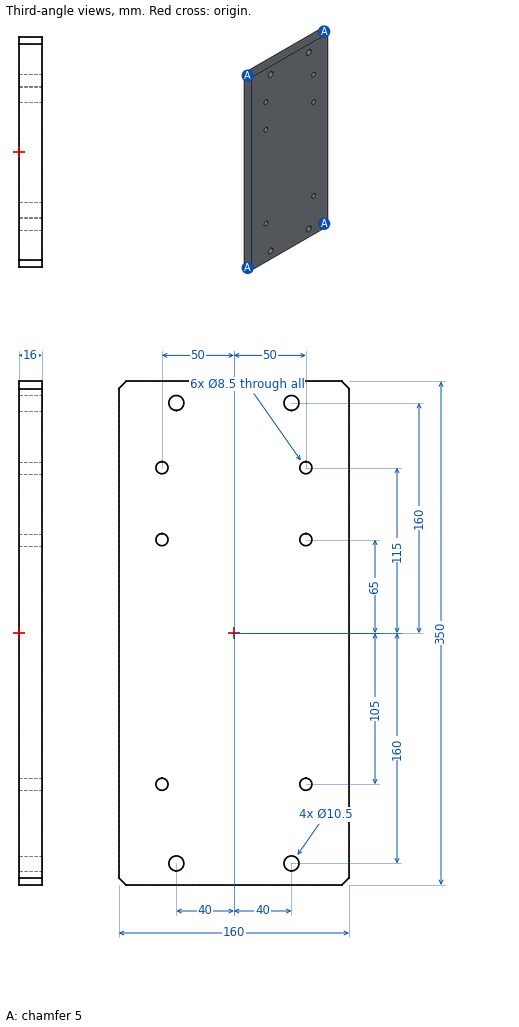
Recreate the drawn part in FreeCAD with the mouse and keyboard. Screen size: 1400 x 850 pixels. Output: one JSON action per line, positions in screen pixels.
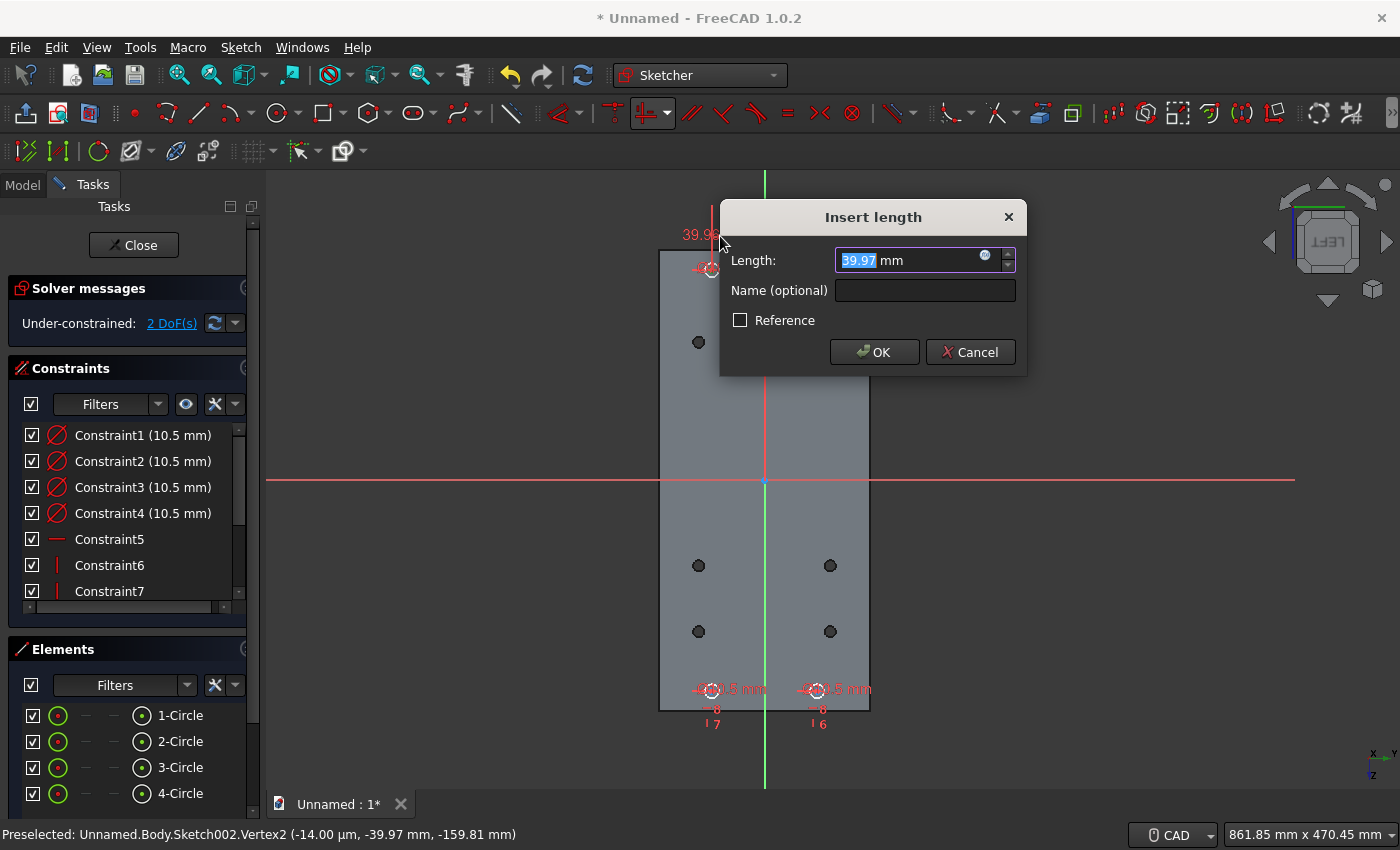
{"action": "type", "text": "40"}
{"action": "key", "text": "Return"}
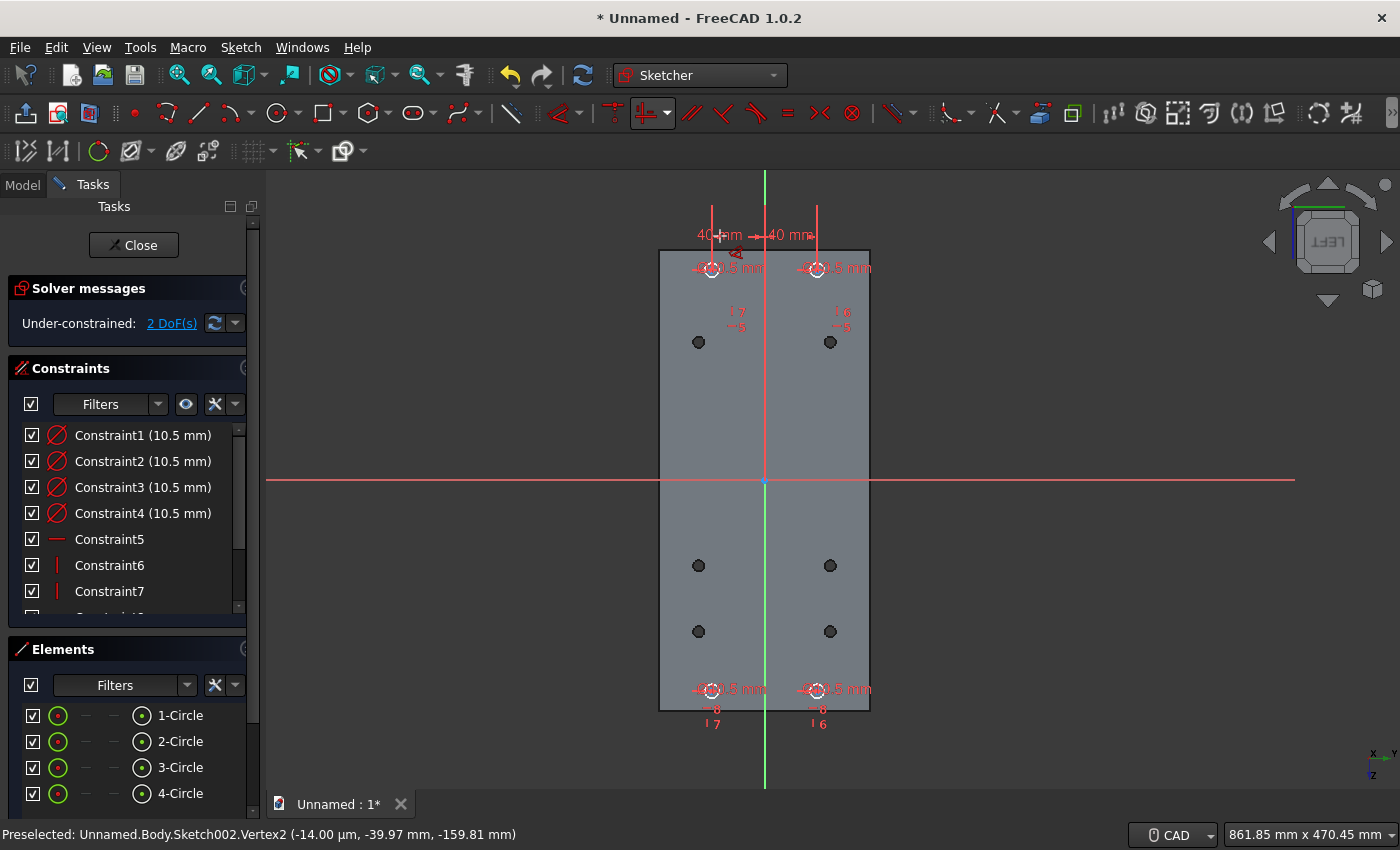
{"action": "left_click", "coordinate": [817, 270]}
{"action": "left_click", "coordinate": [851, 375]}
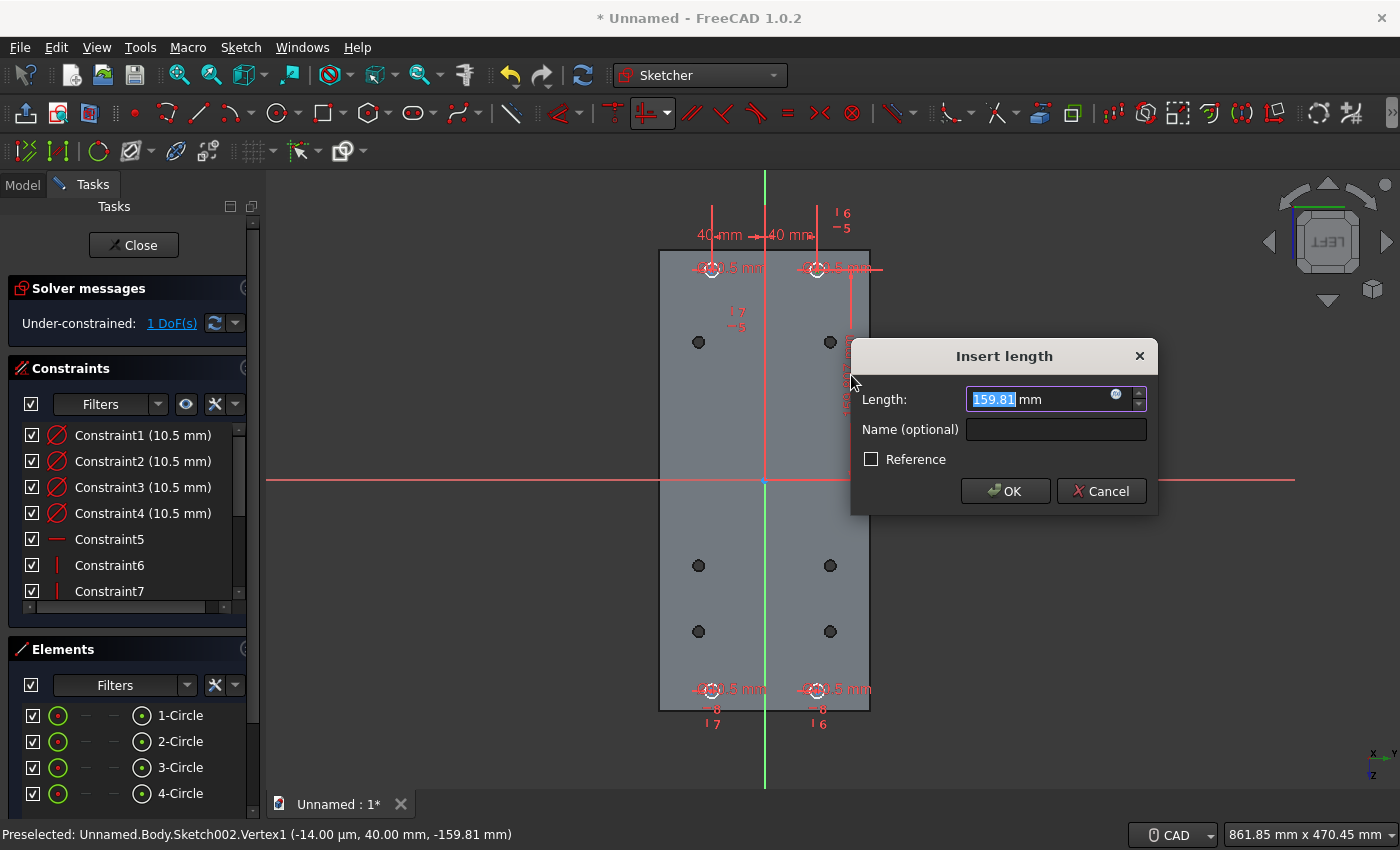
{"action": "type", "text": "160"}
{"action": "key", "text": "Return"}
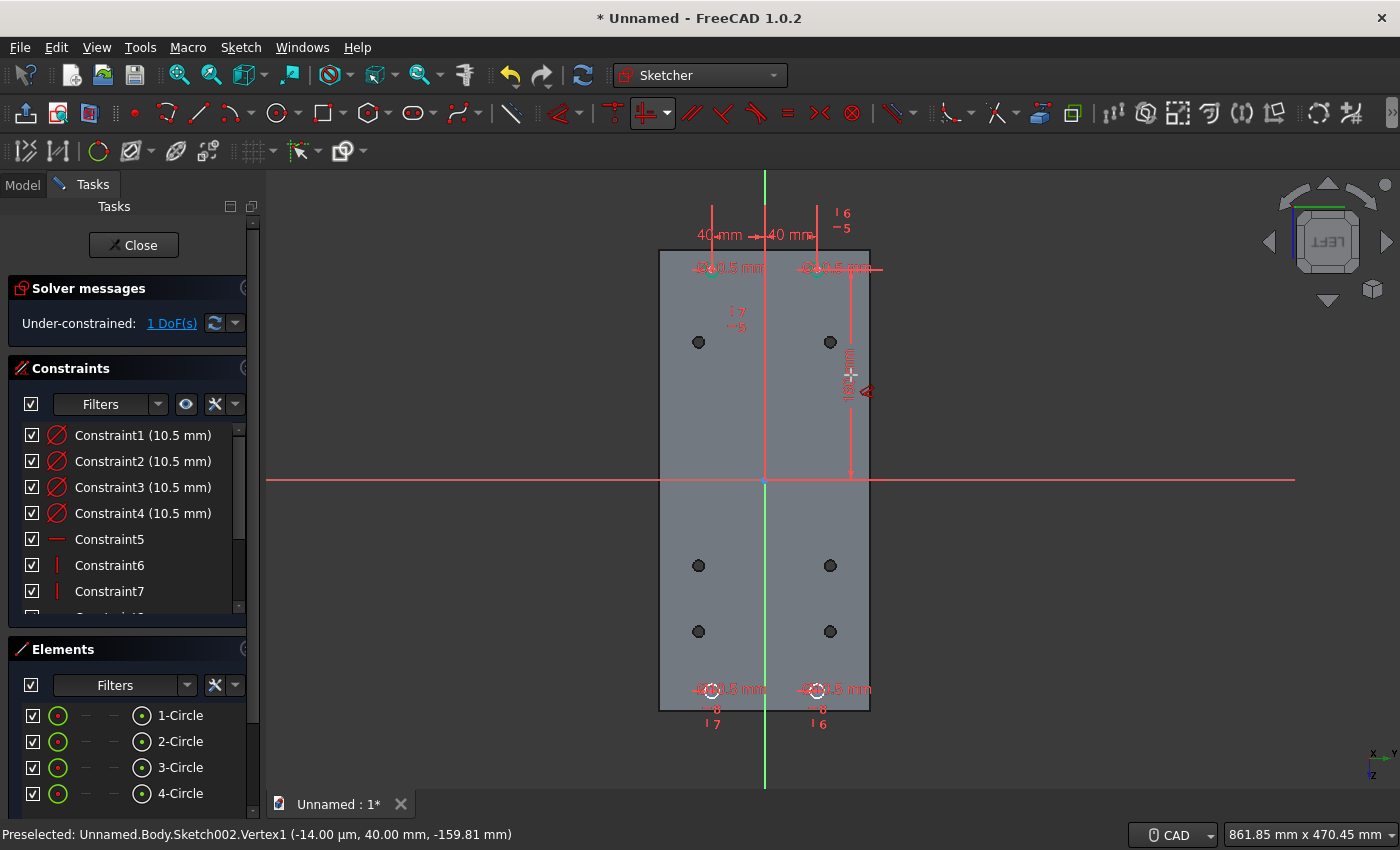
{"action": "left_click", "coordinate": [817, 691]}
{"action": "left_click", "coordinate": [851, 586]}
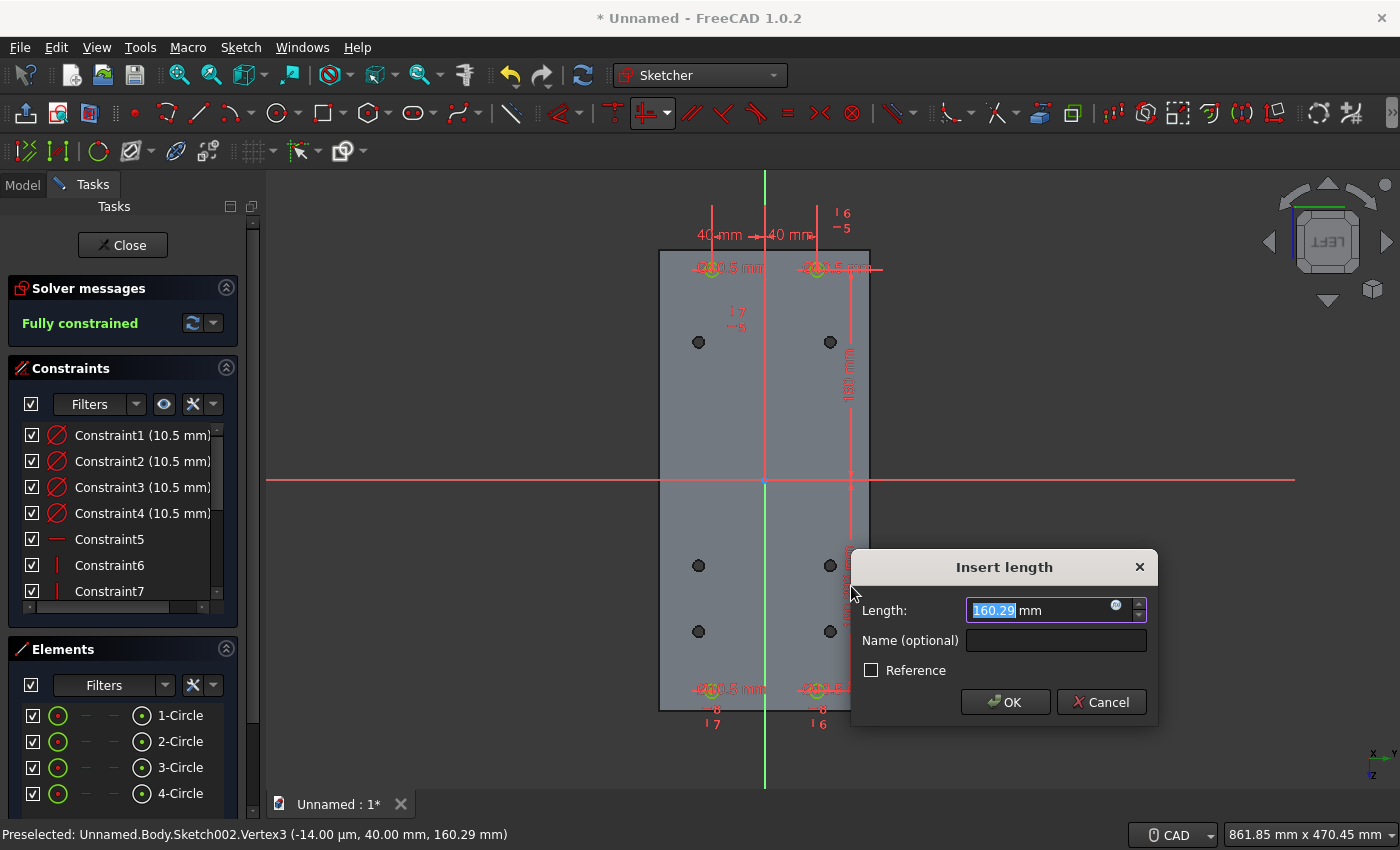
{"action": "type", "text": "160"}
{"action": "key", "text": "Return"}
{"action": "key", "text": "Escape"}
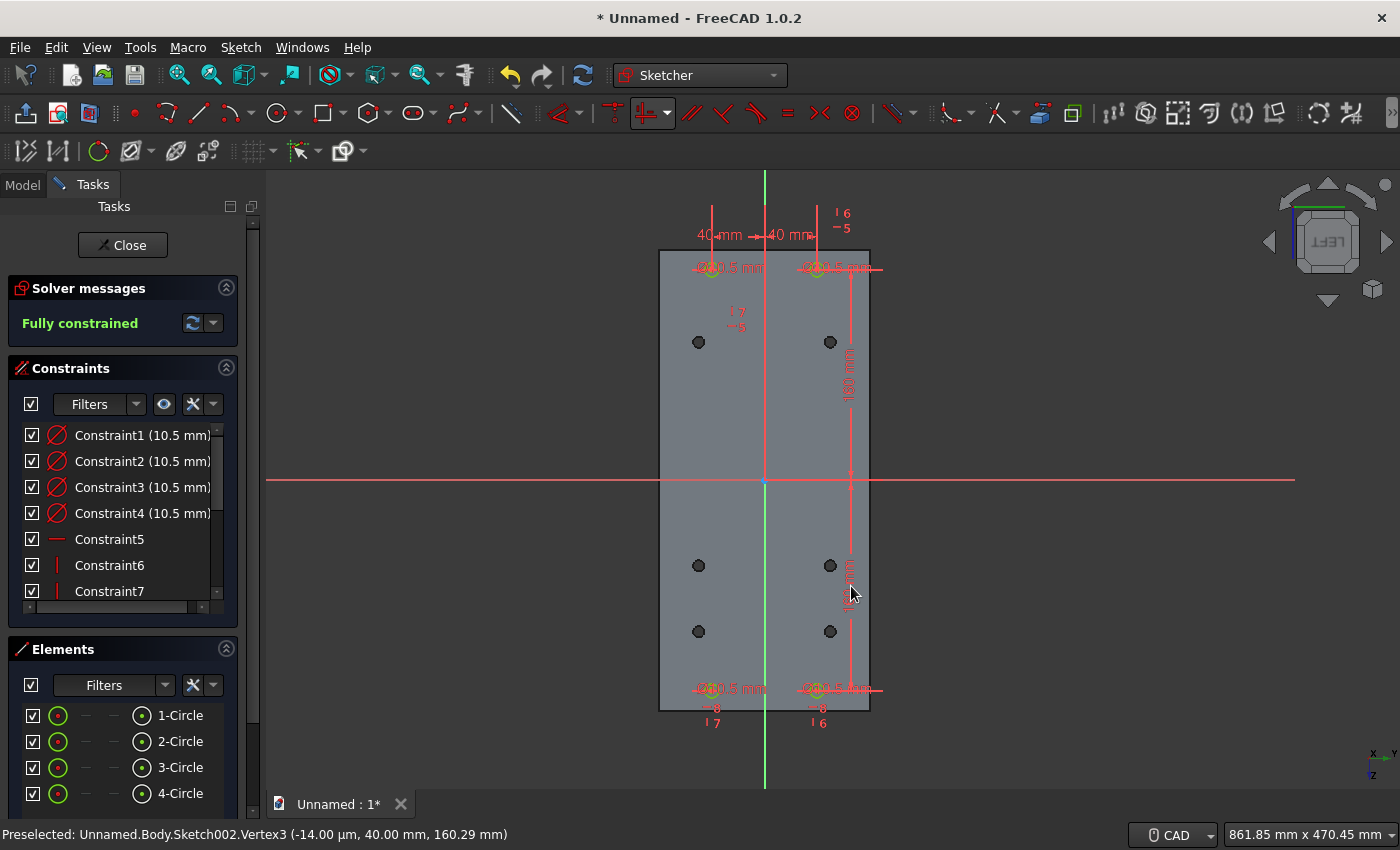
{"action": "left_click", "coordinate": [123, 245]}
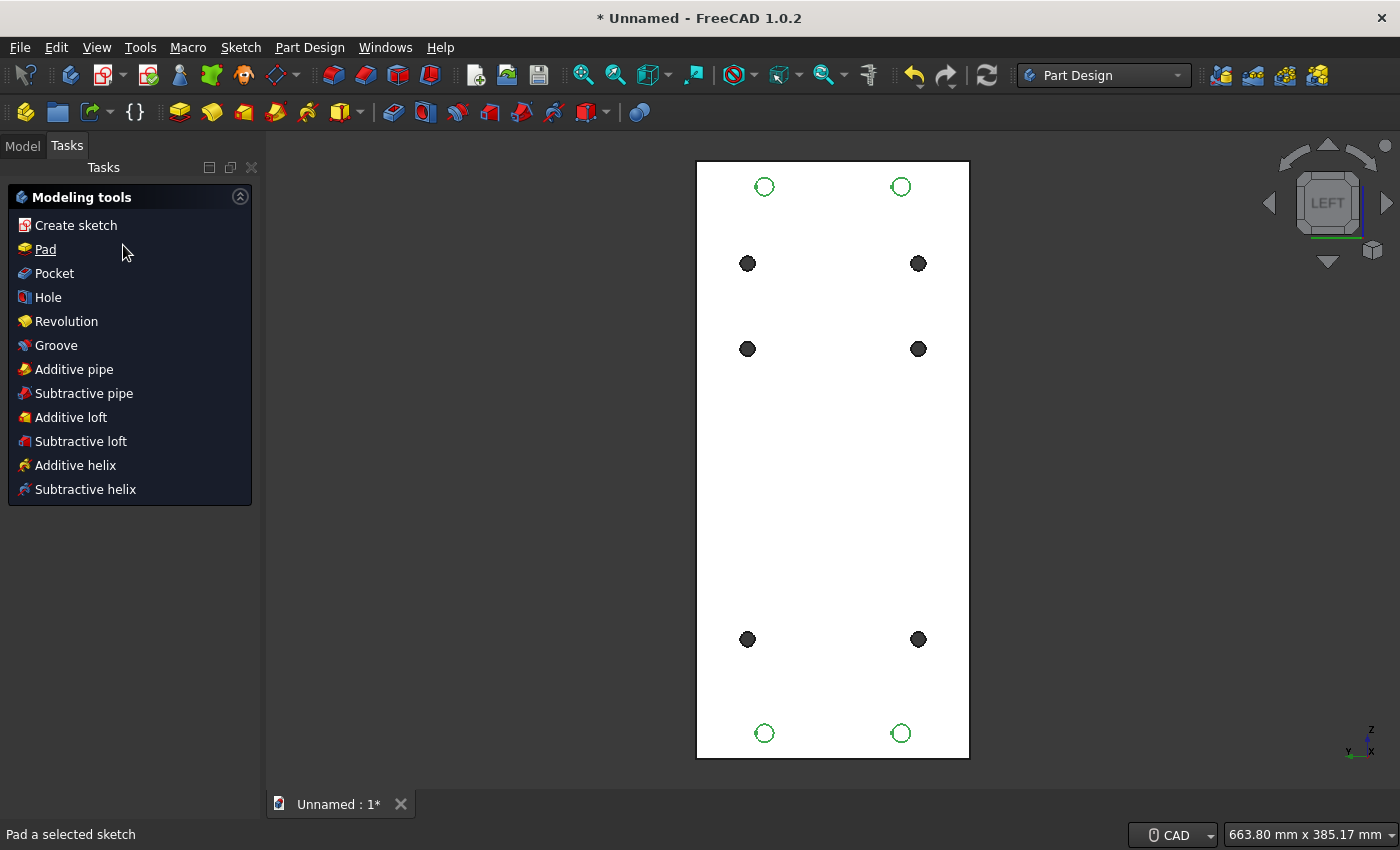
{"action": "left_click", "coordinate": [394, 112]}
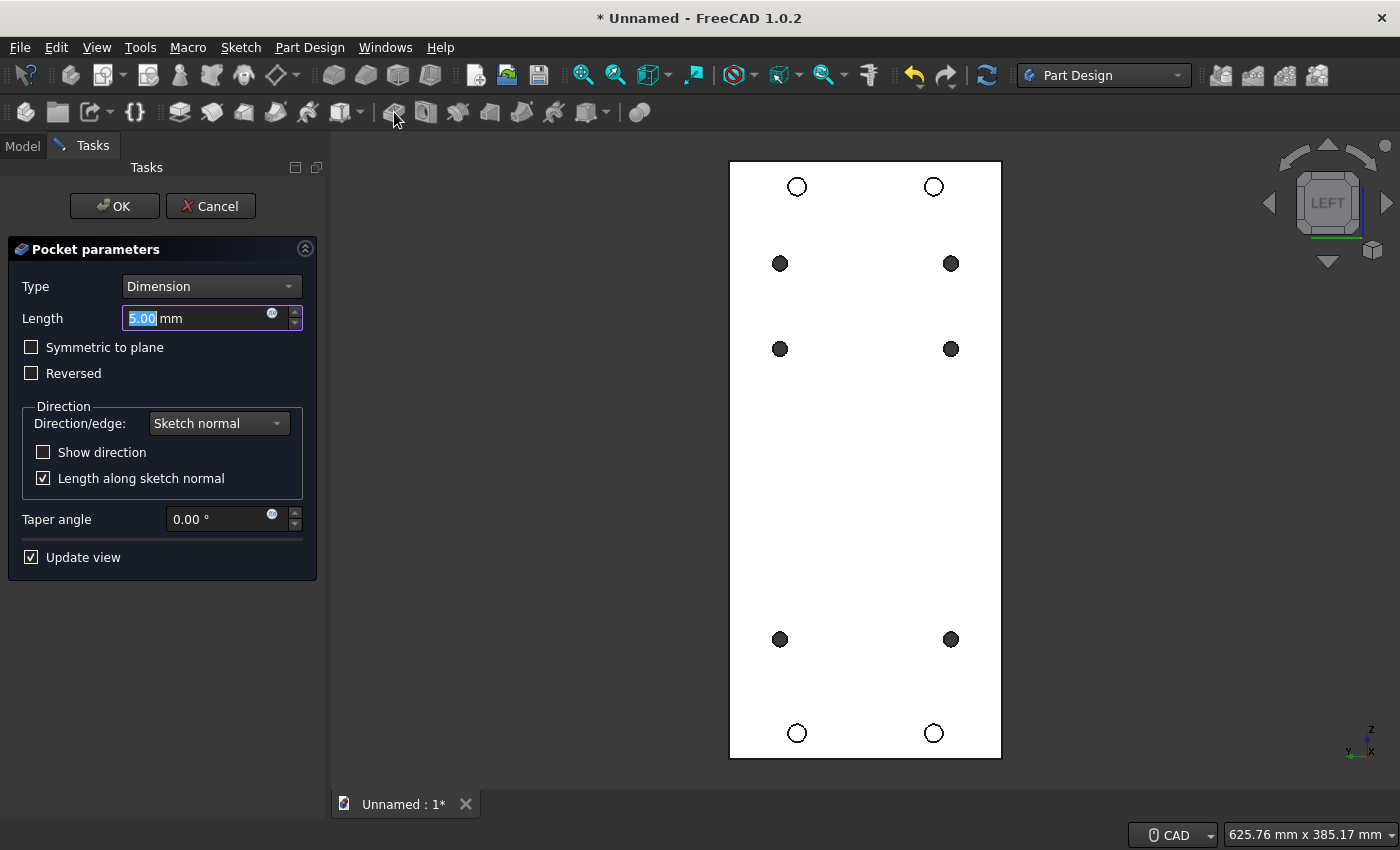
{"action": "left_click", "coordinate": [212, 286]}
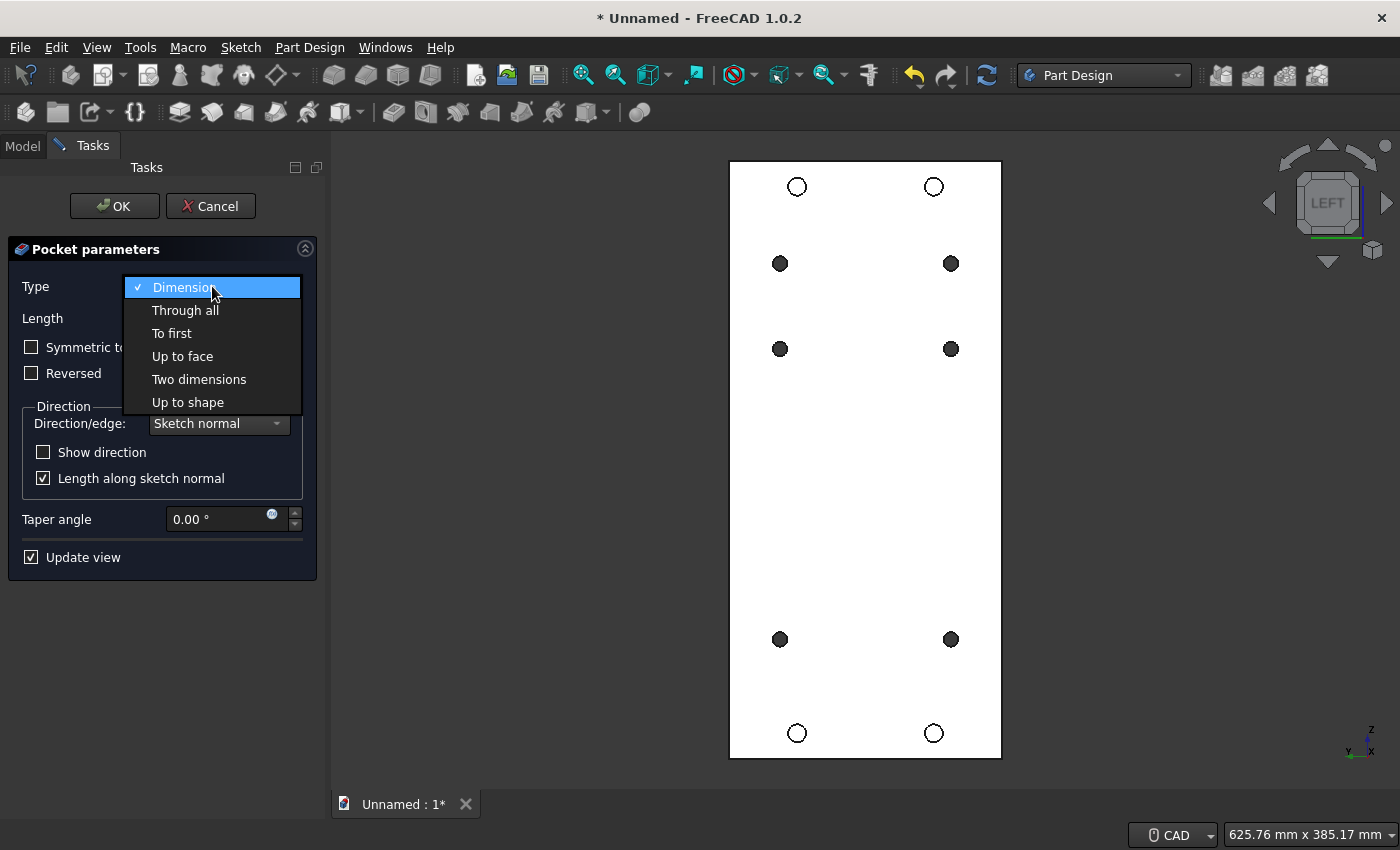
{"action": "left_click", "coordinate": [212, 310]}